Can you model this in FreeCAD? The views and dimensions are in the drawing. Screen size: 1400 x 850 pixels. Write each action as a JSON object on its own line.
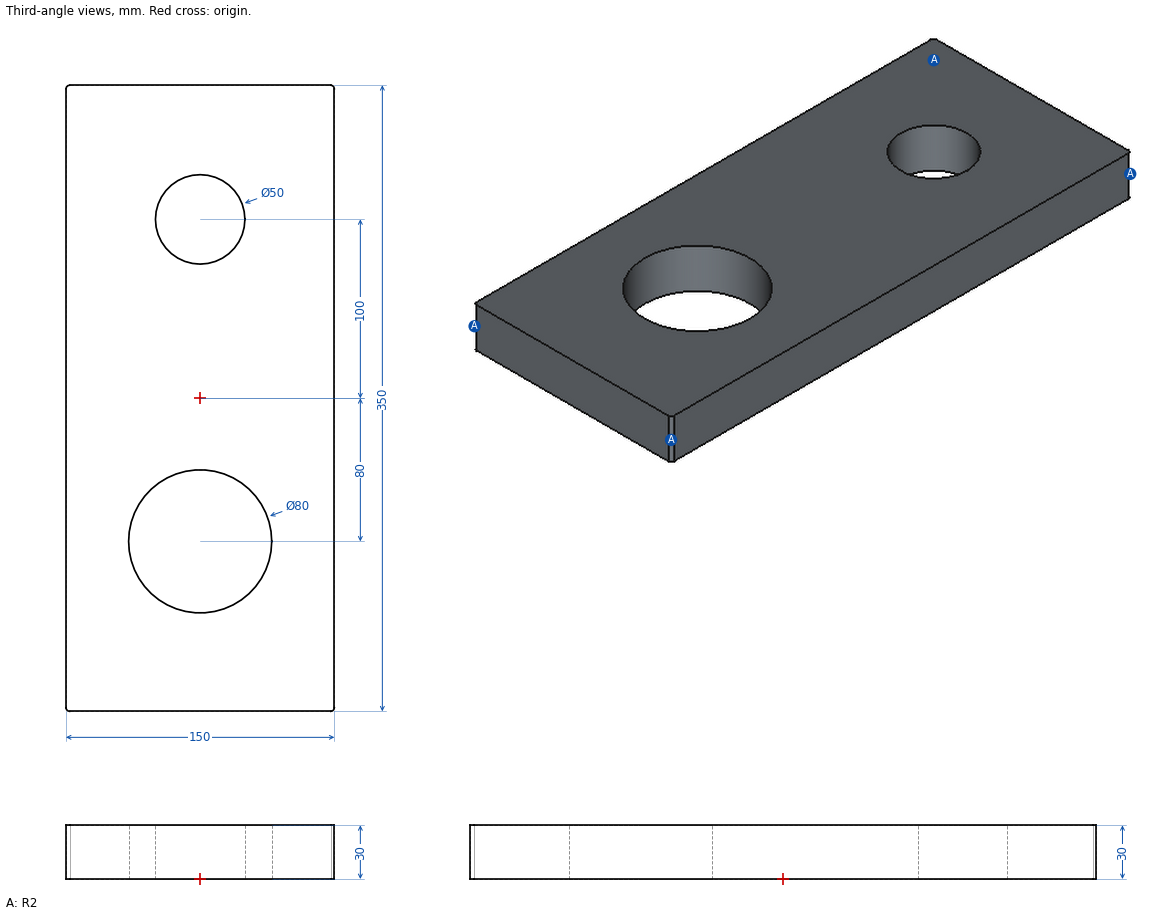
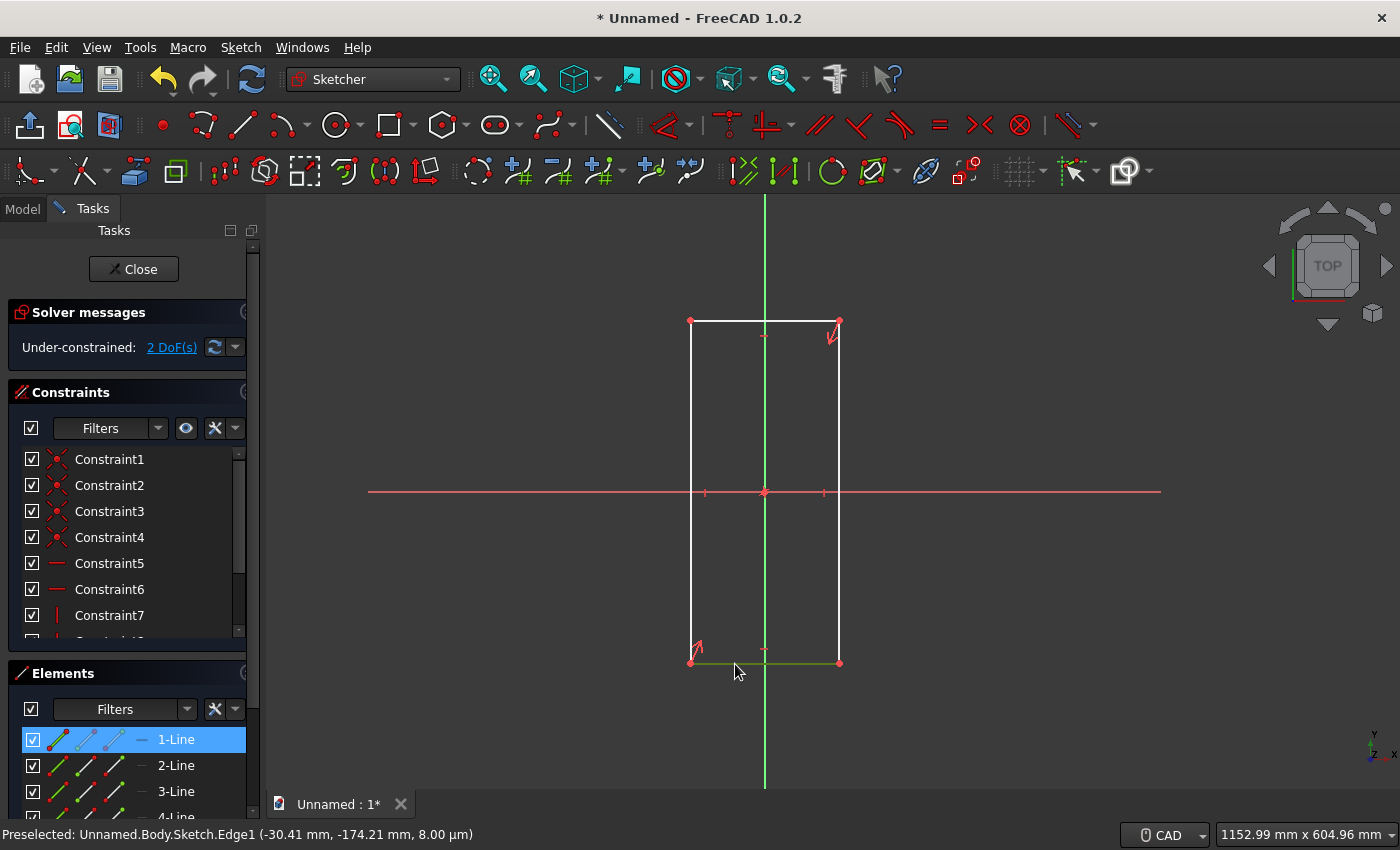
{"action": "key", "text": "l"}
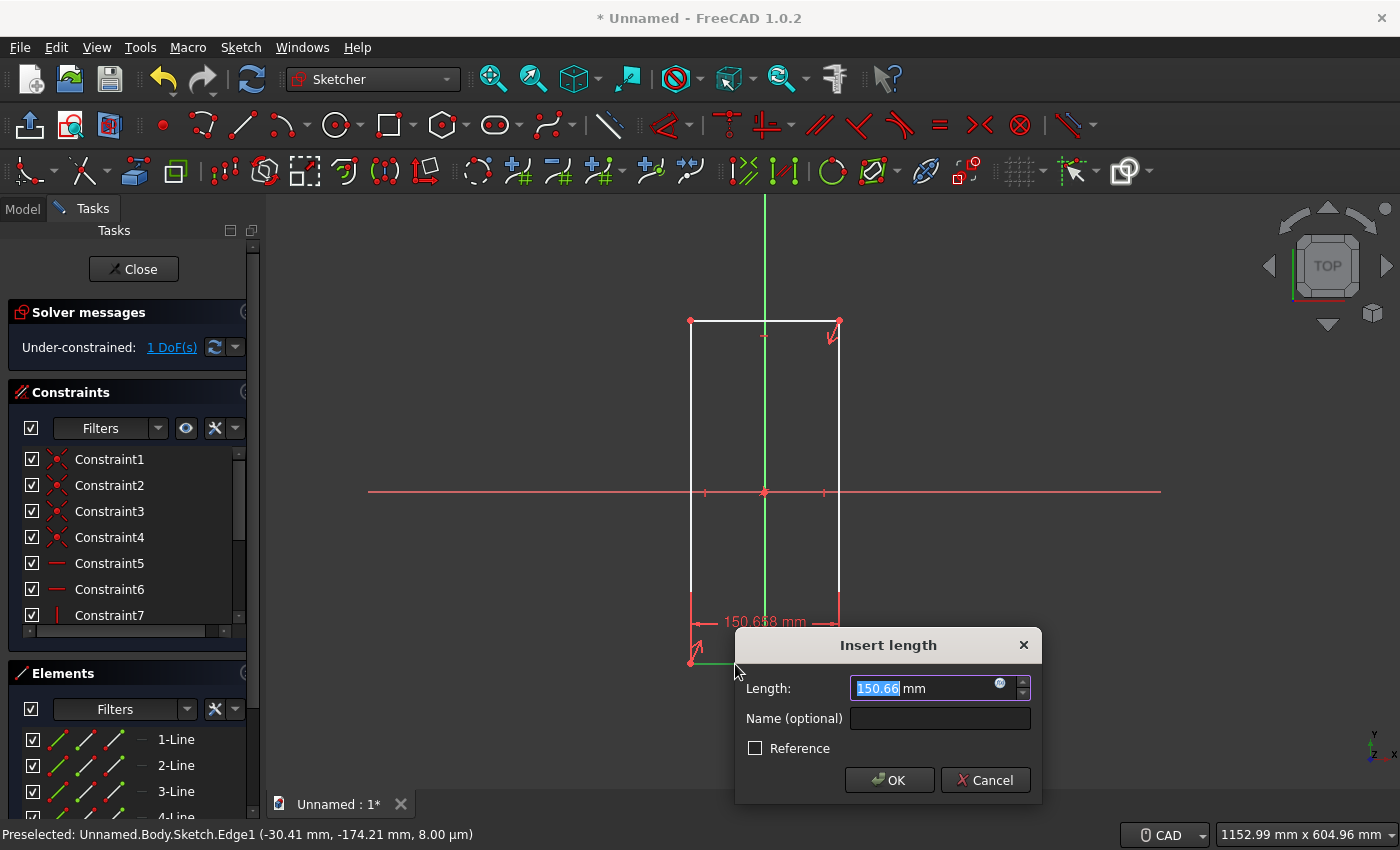
{"action": "type", "text": "150"}
{"action": "key", "text": "Return"}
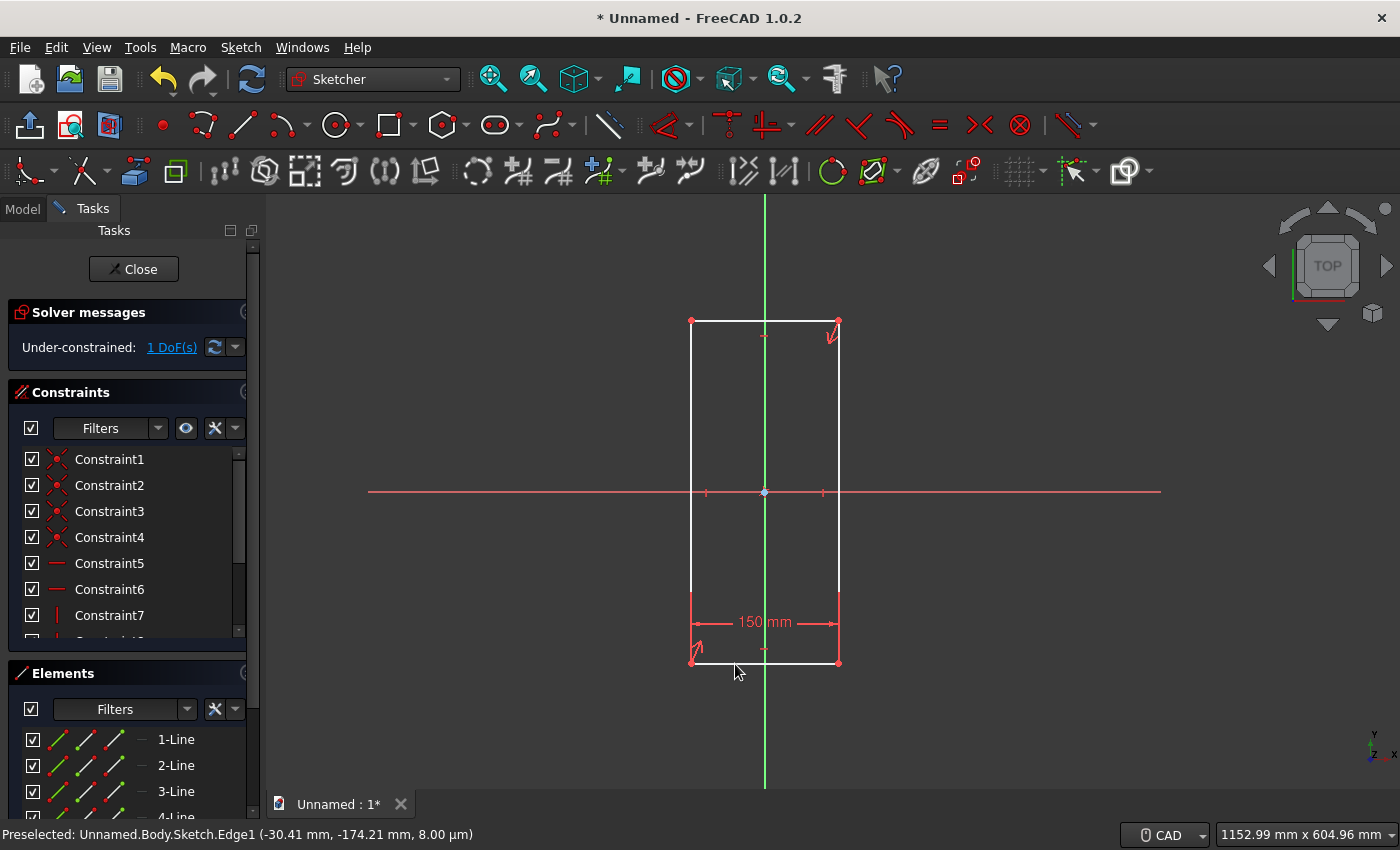
{"action": "left_click", "coordinate": [839, 561]}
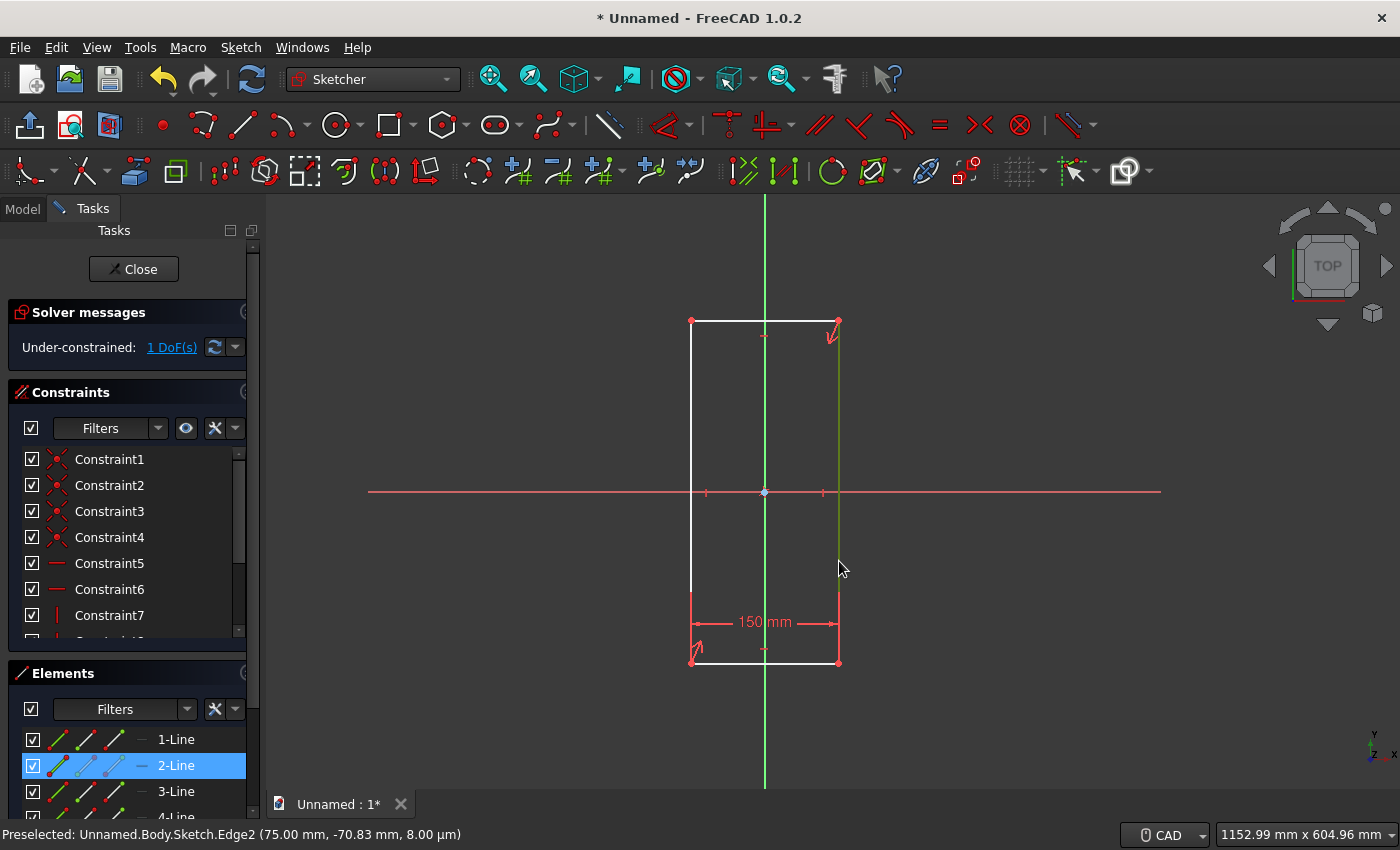
{"action": "left_click", "coordinate": [692, 126]}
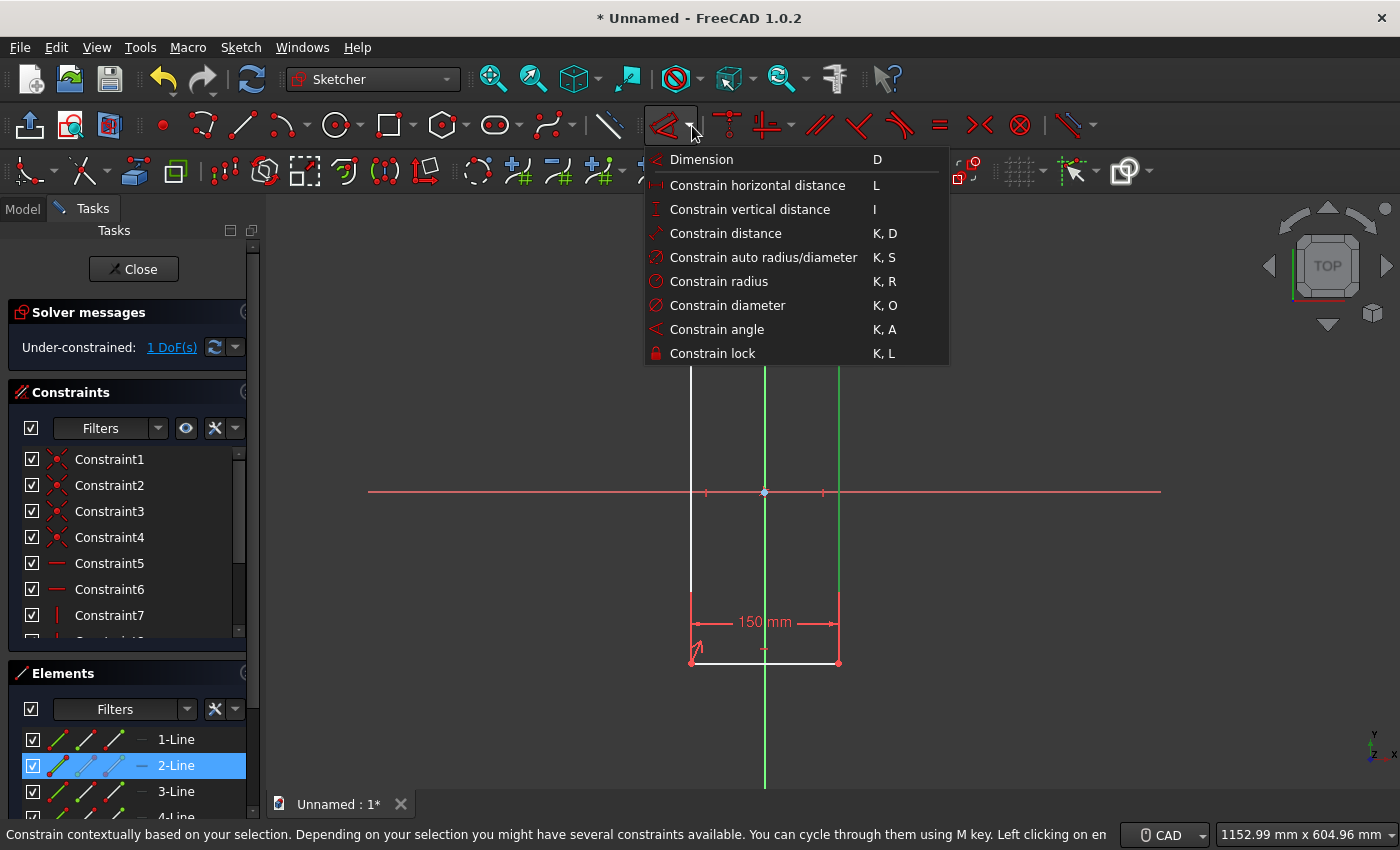
{"action": "left_click", "coordinate": [797, 209]}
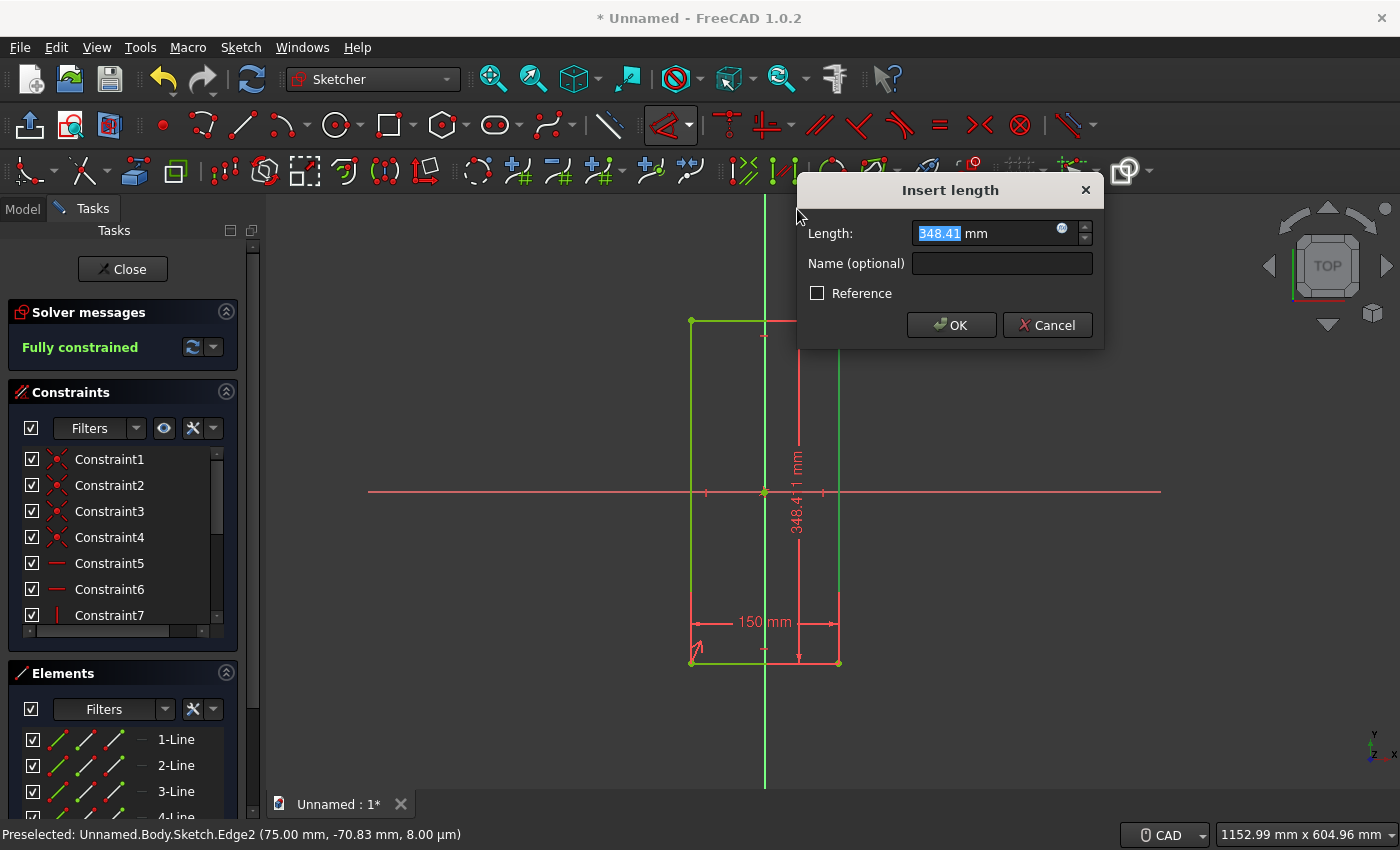
{"action": "type", "text": "350"}
{"action": "key", "text": "Return"}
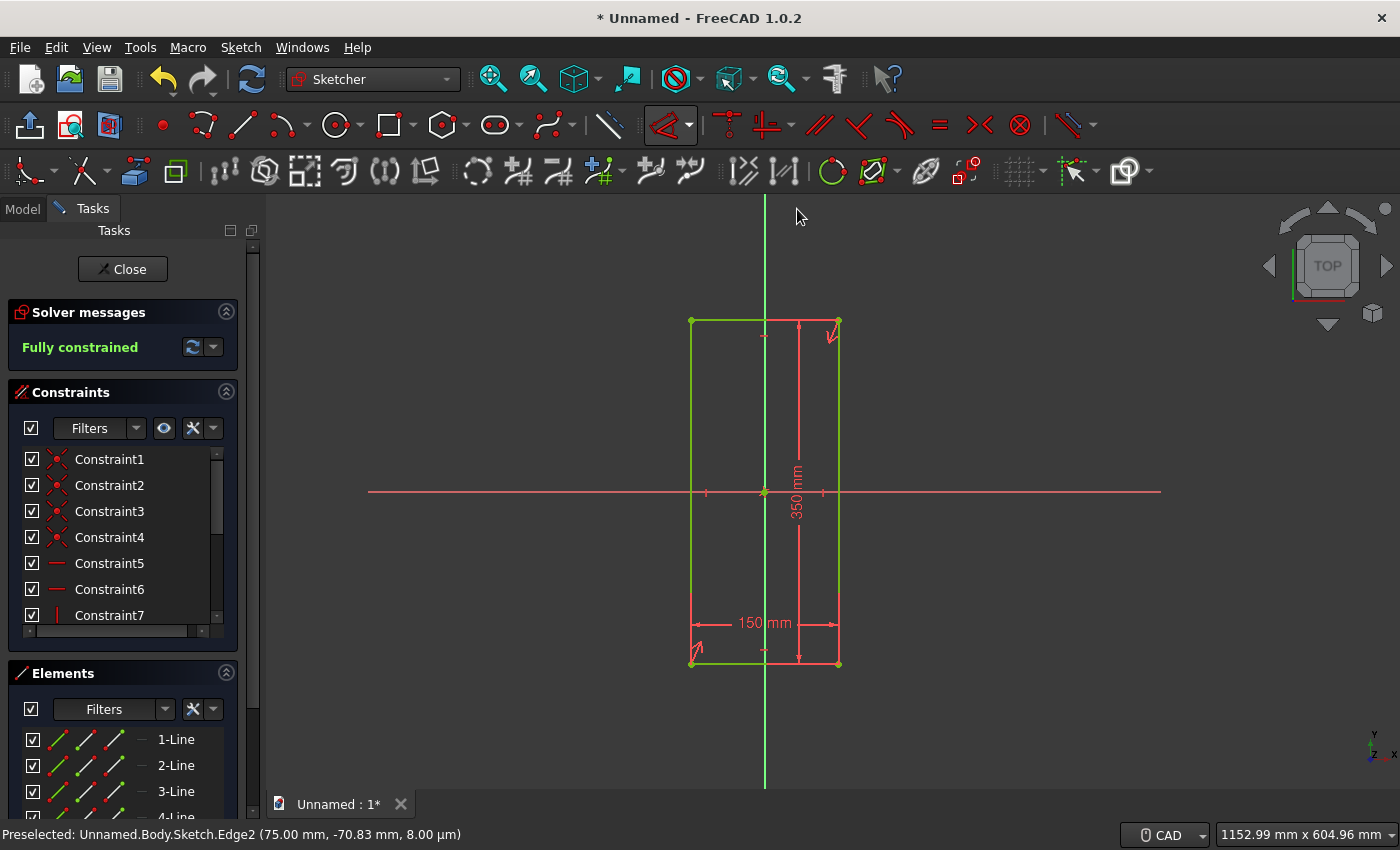
{"action": "left_click", "coordinate": [123, 269]}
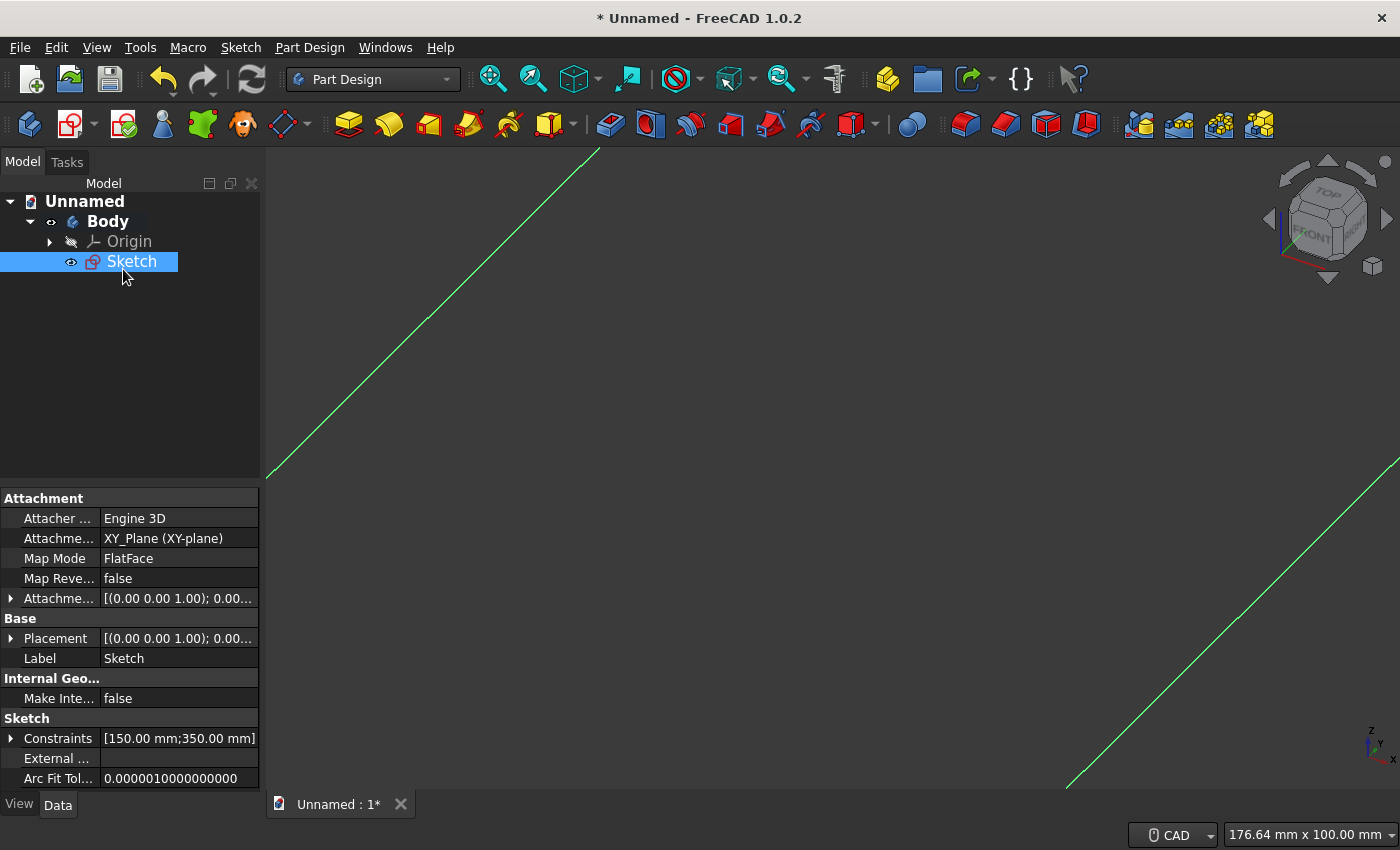
{"action": "left_click", "coordinate": [350, 124]}